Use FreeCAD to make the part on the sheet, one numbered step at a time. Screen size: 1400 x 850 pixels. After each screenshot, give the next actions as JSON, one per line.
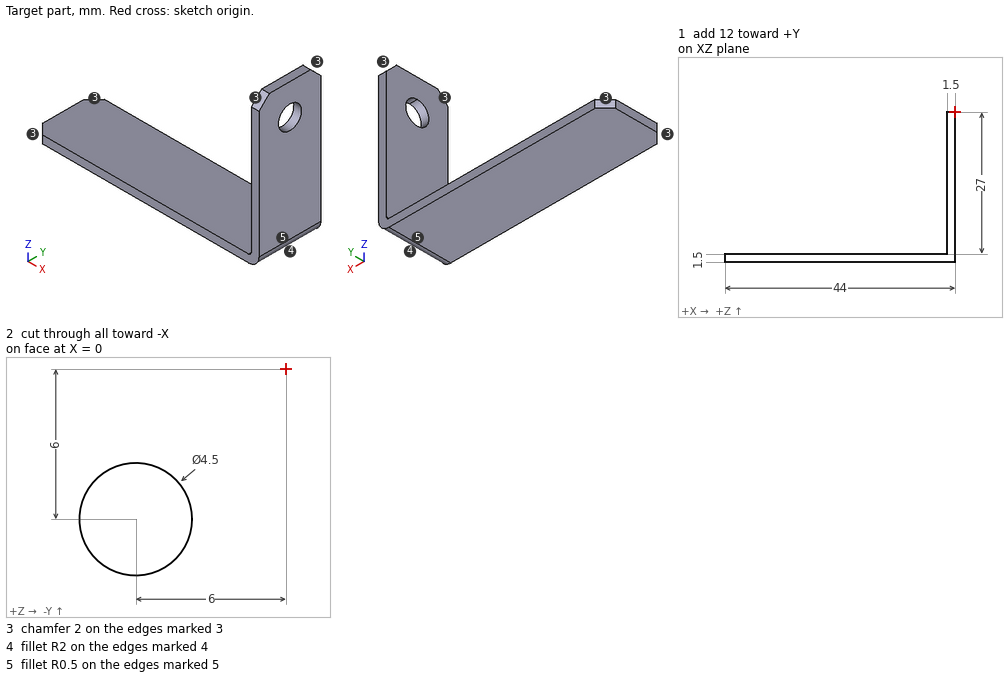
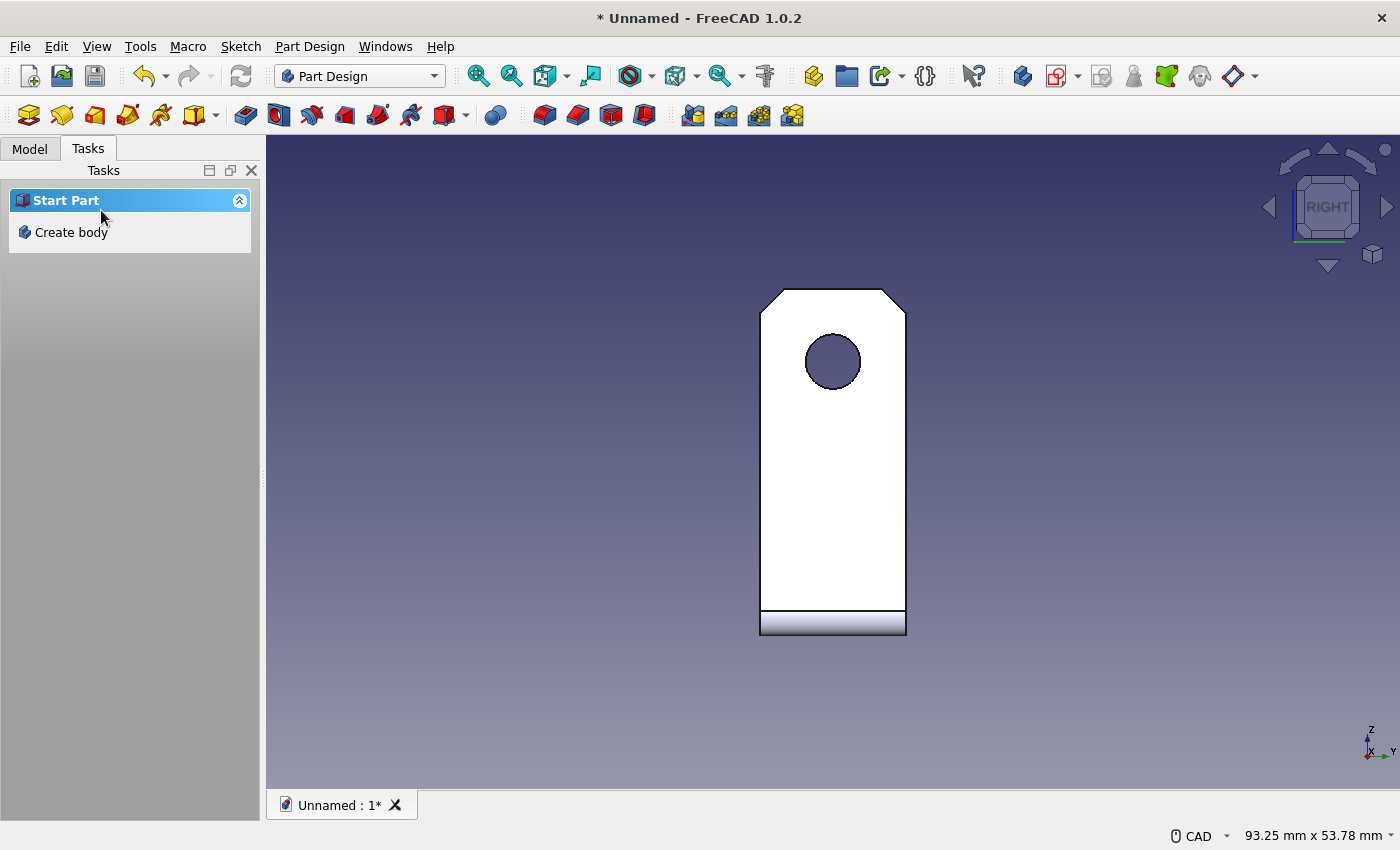
{"action": "key", "text": "5"}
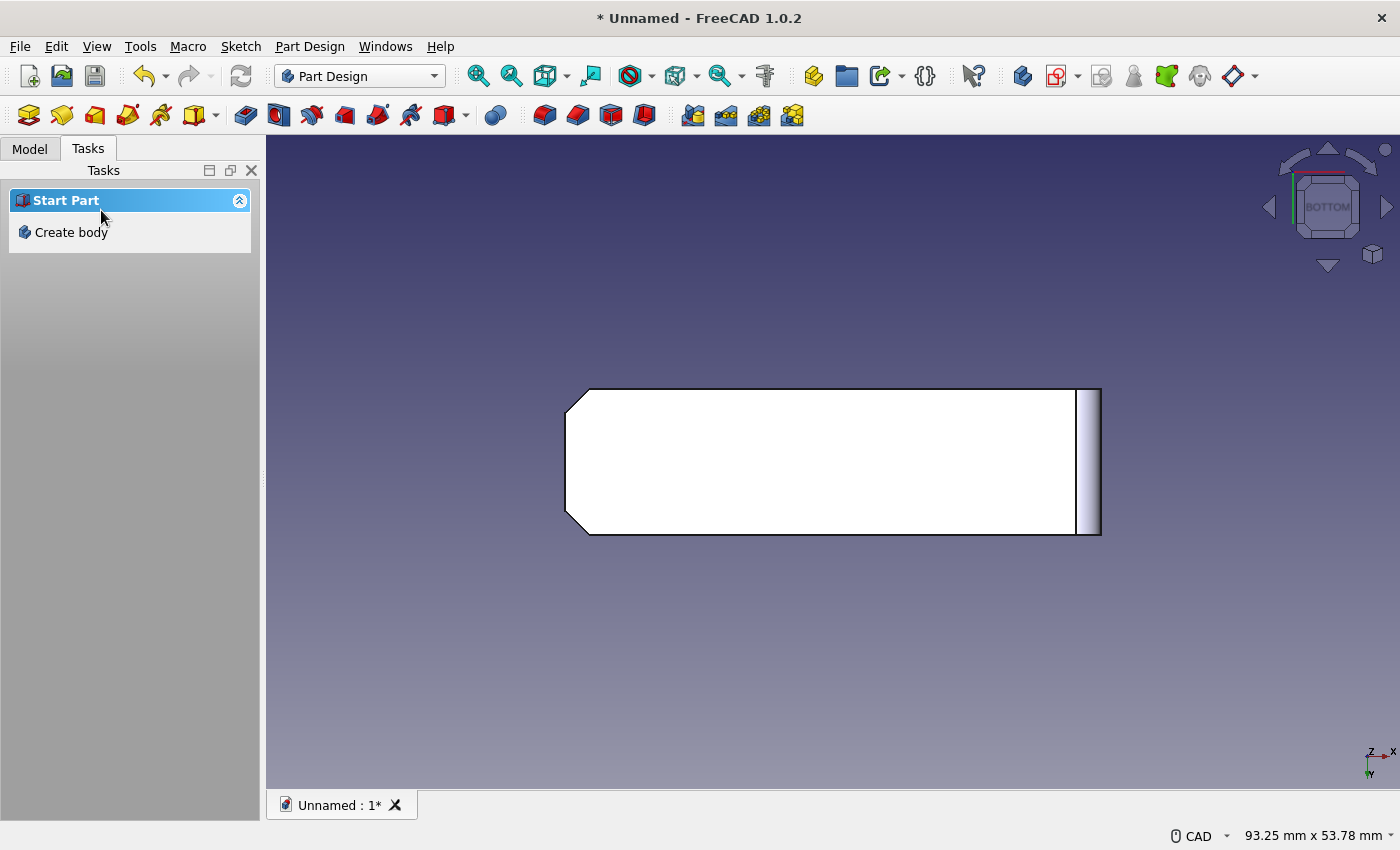
{"action": "key", "text": "4"}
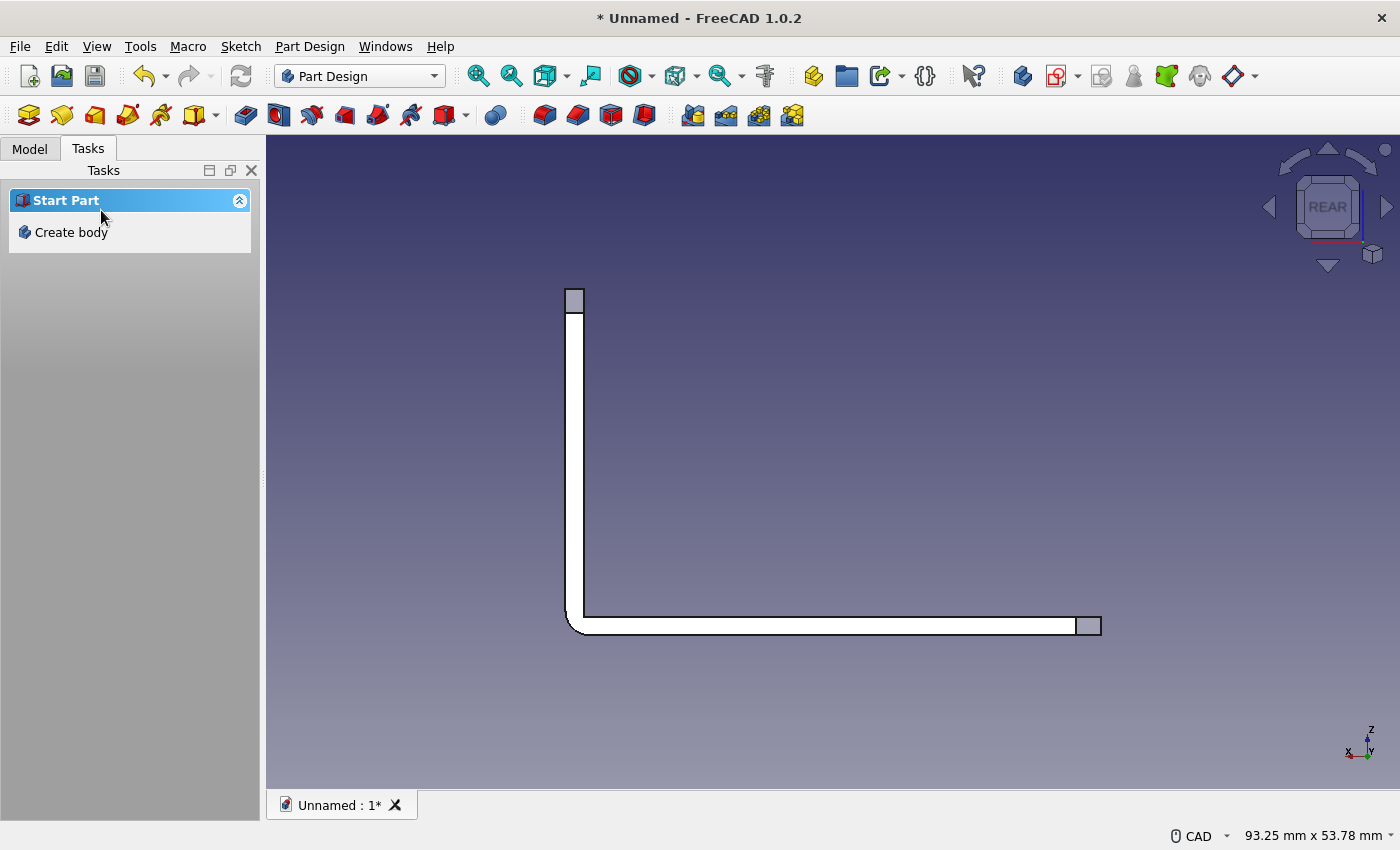
{"action": "key", "text": "6"}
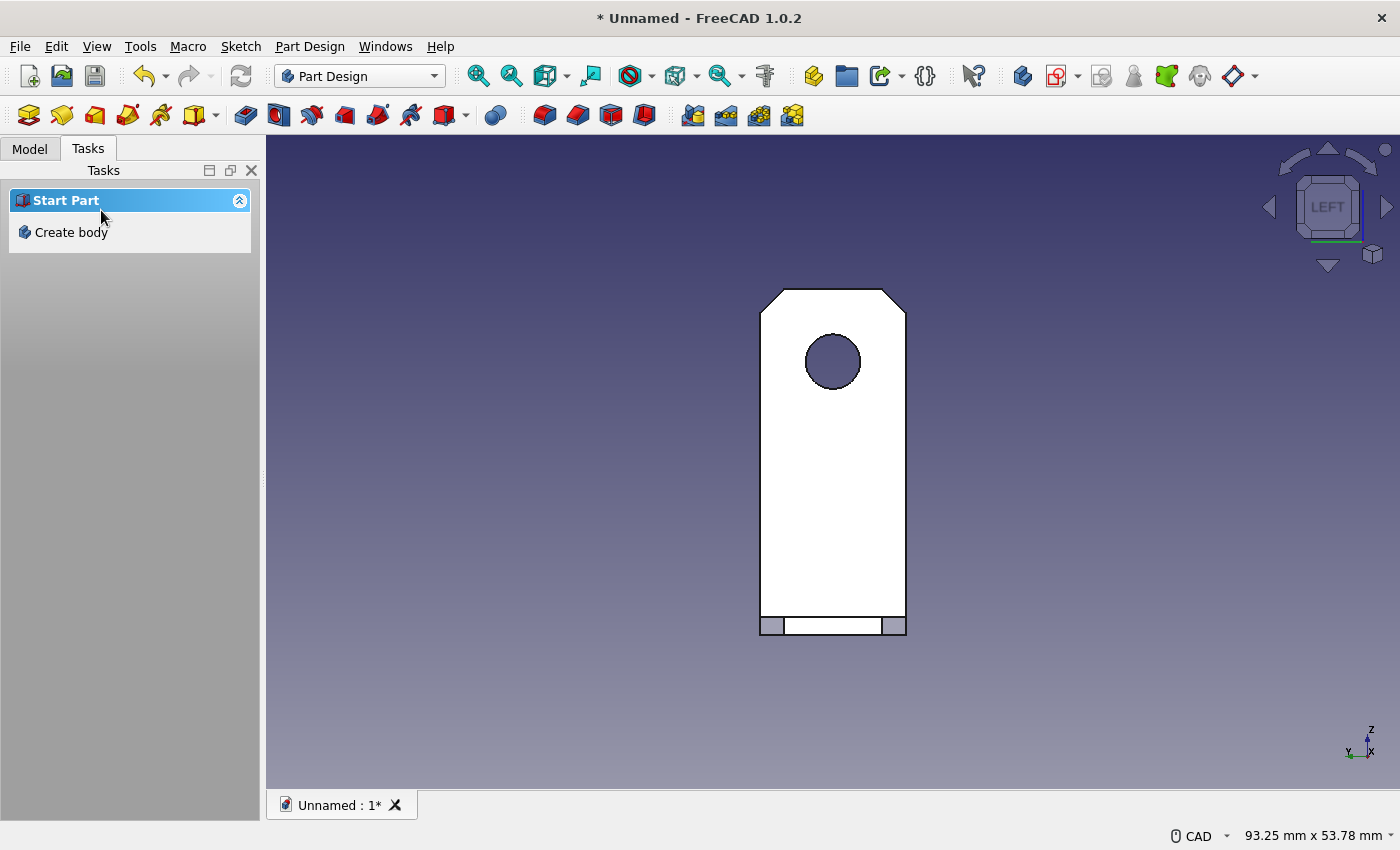
{"action": "key", "text": "v 3"}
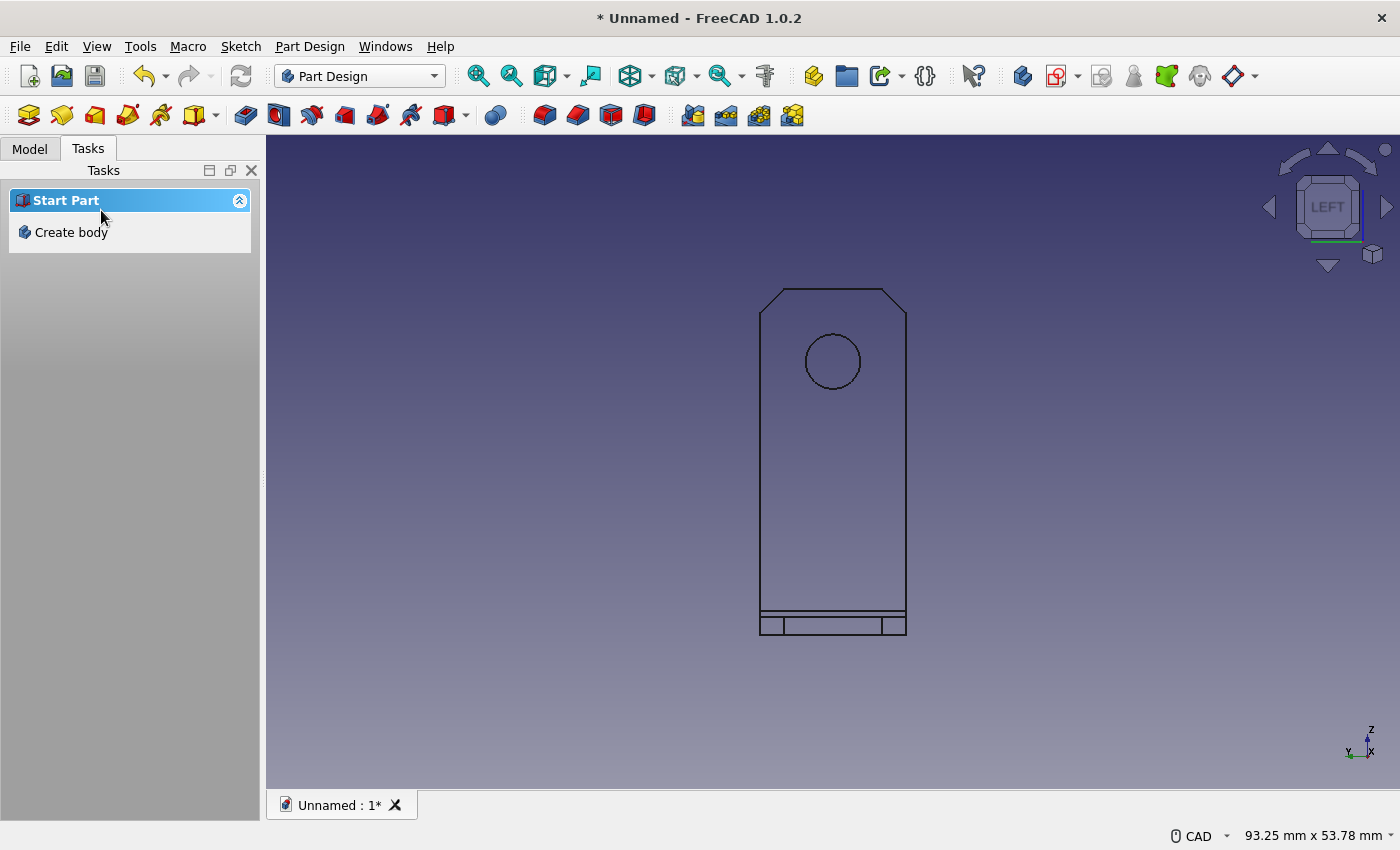
{"action": "key", "text": "0"}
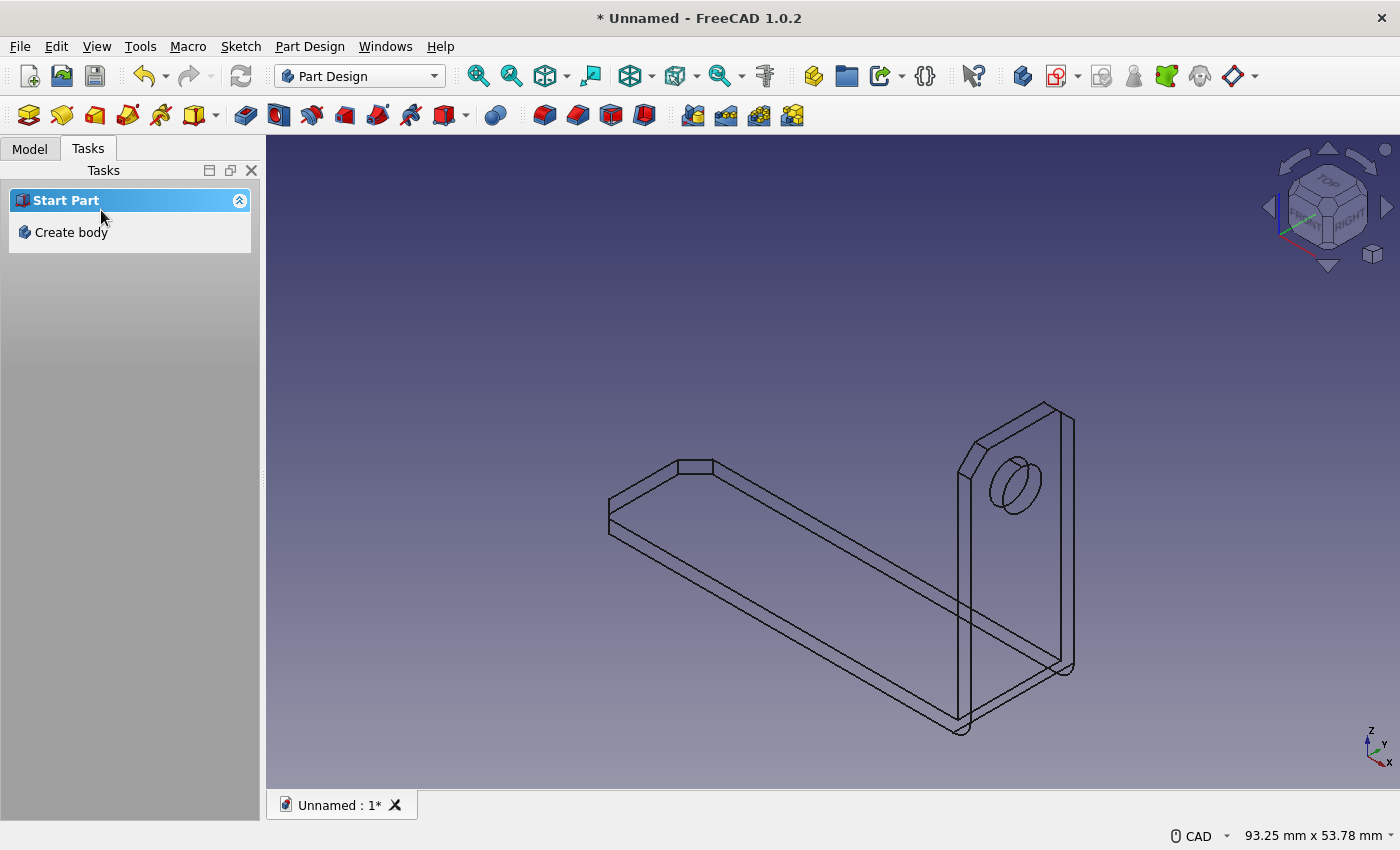
{"action": "left_click", "coordinate": [1009, 689]}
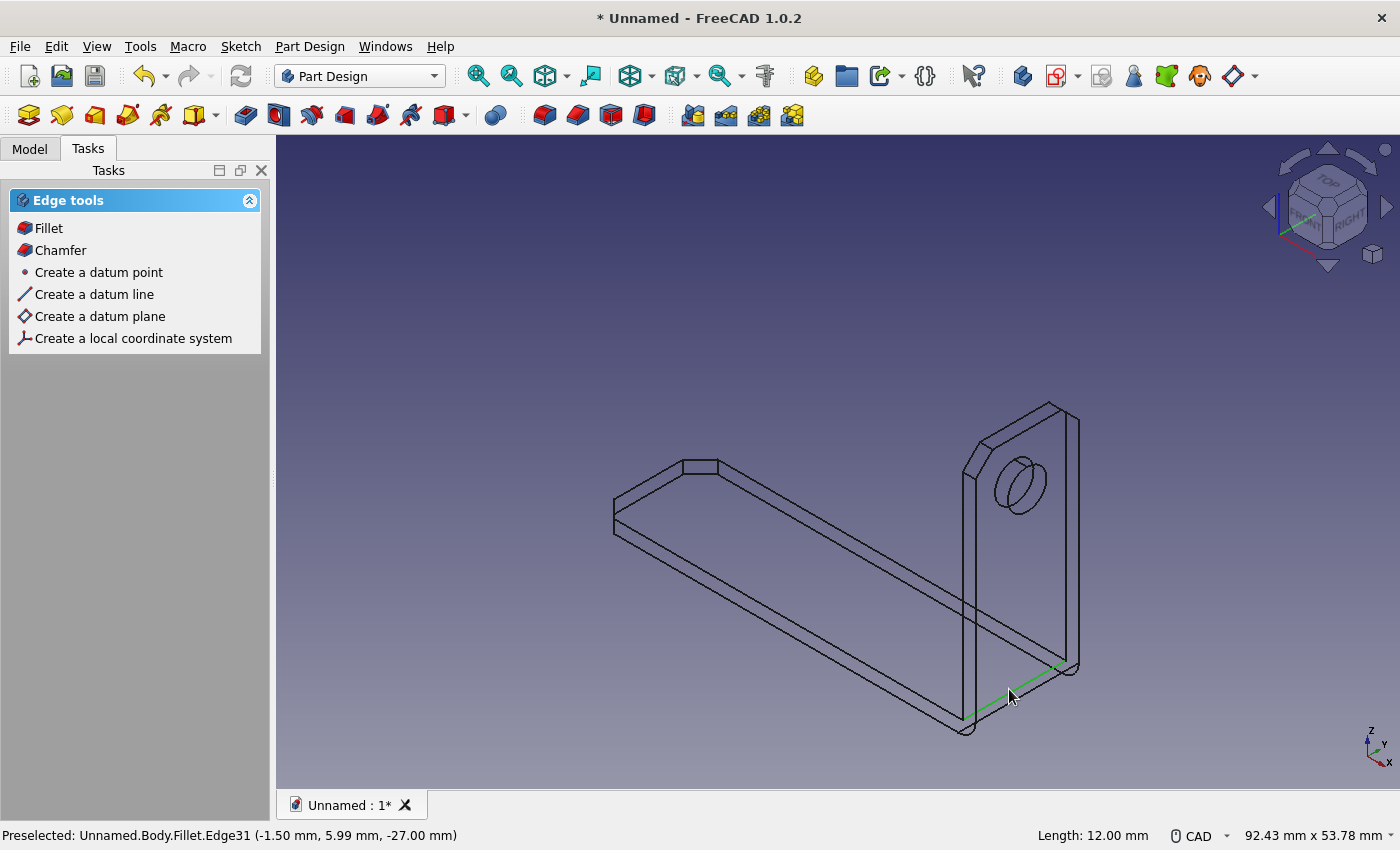
{"action": "key", "text": "v 1"}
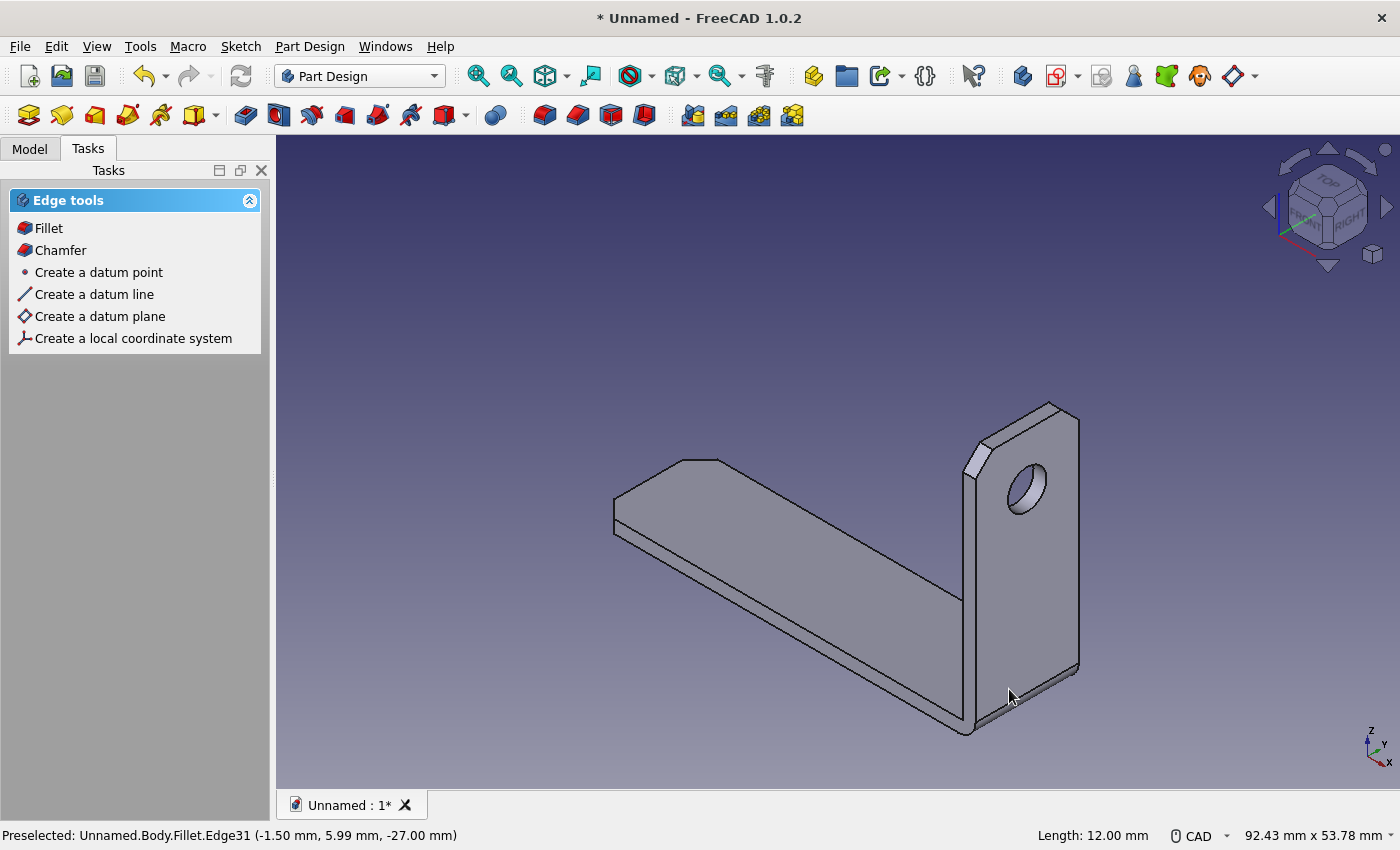
{"action": "left_click", "coordinate": [545, 116]}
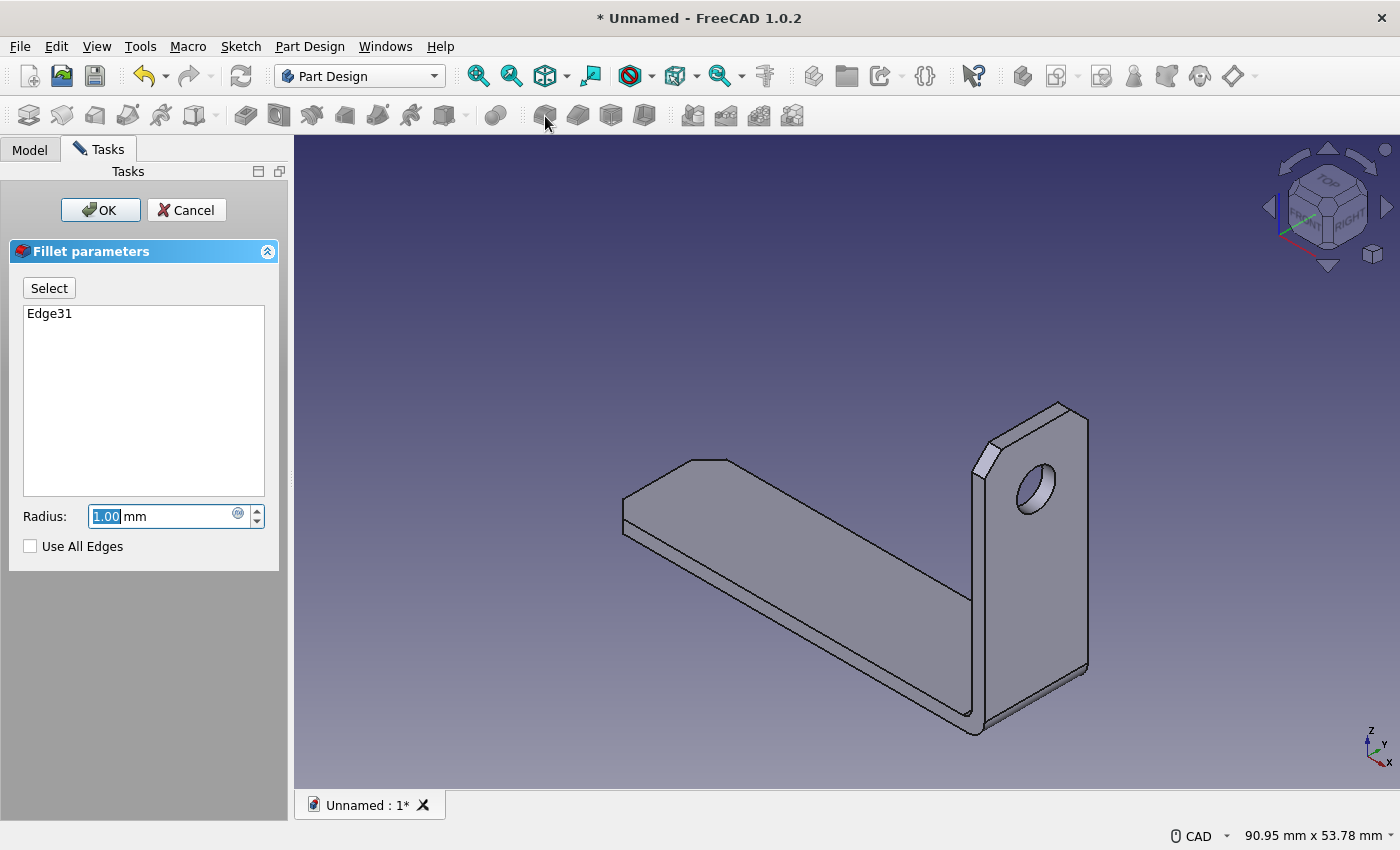
{"action": "type", "text": "0.5"}
{"action": "key", "text": "Tab"}